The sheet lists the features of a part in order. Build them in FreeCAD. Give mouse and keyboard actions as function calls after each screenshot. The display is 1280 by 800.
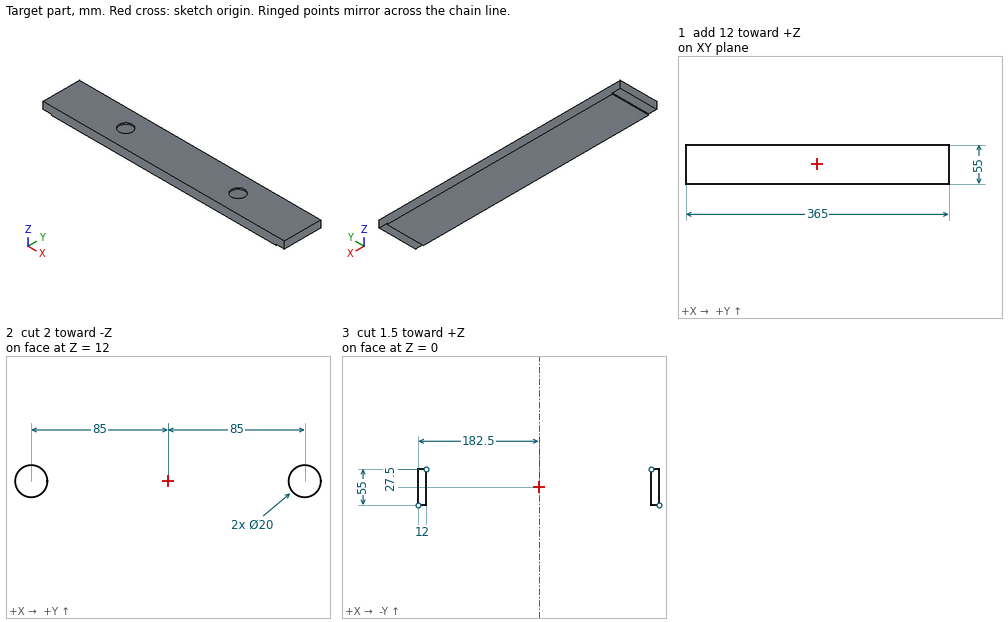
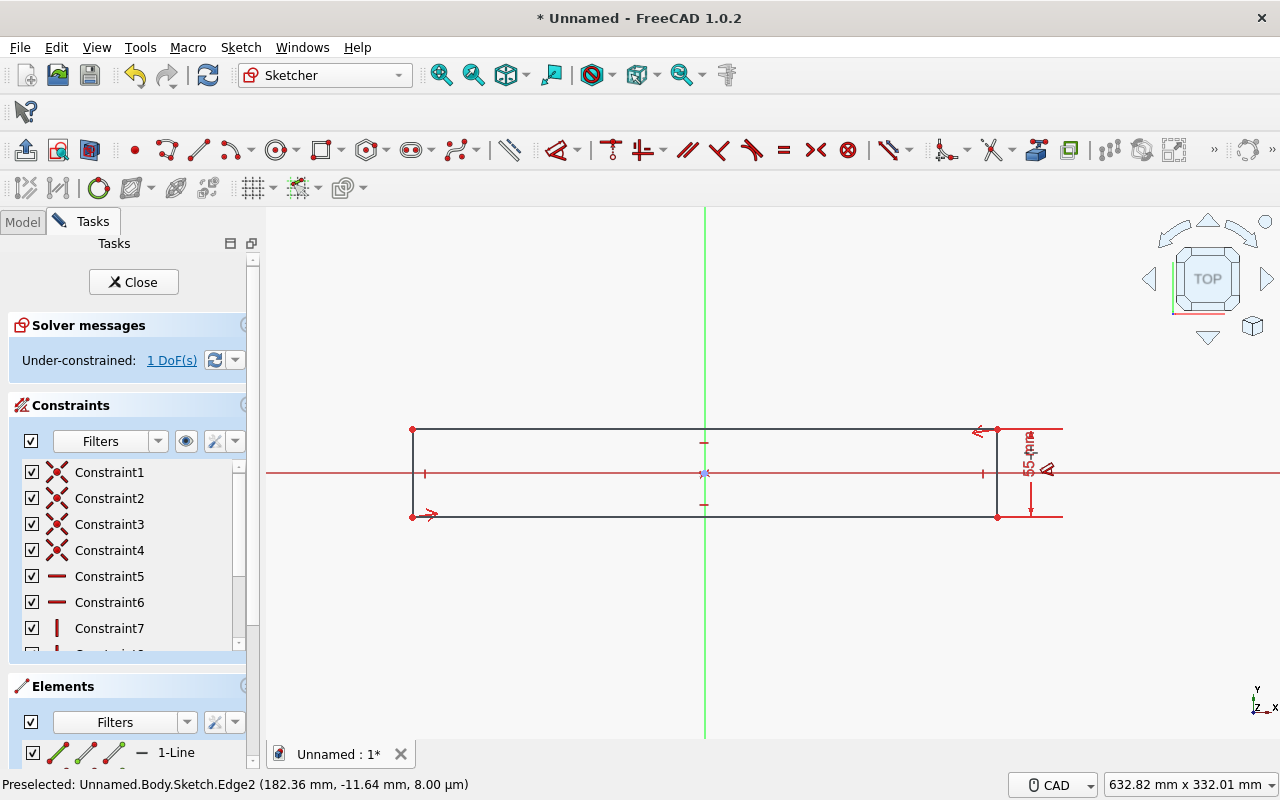
click(588, 517)
click(570, 551)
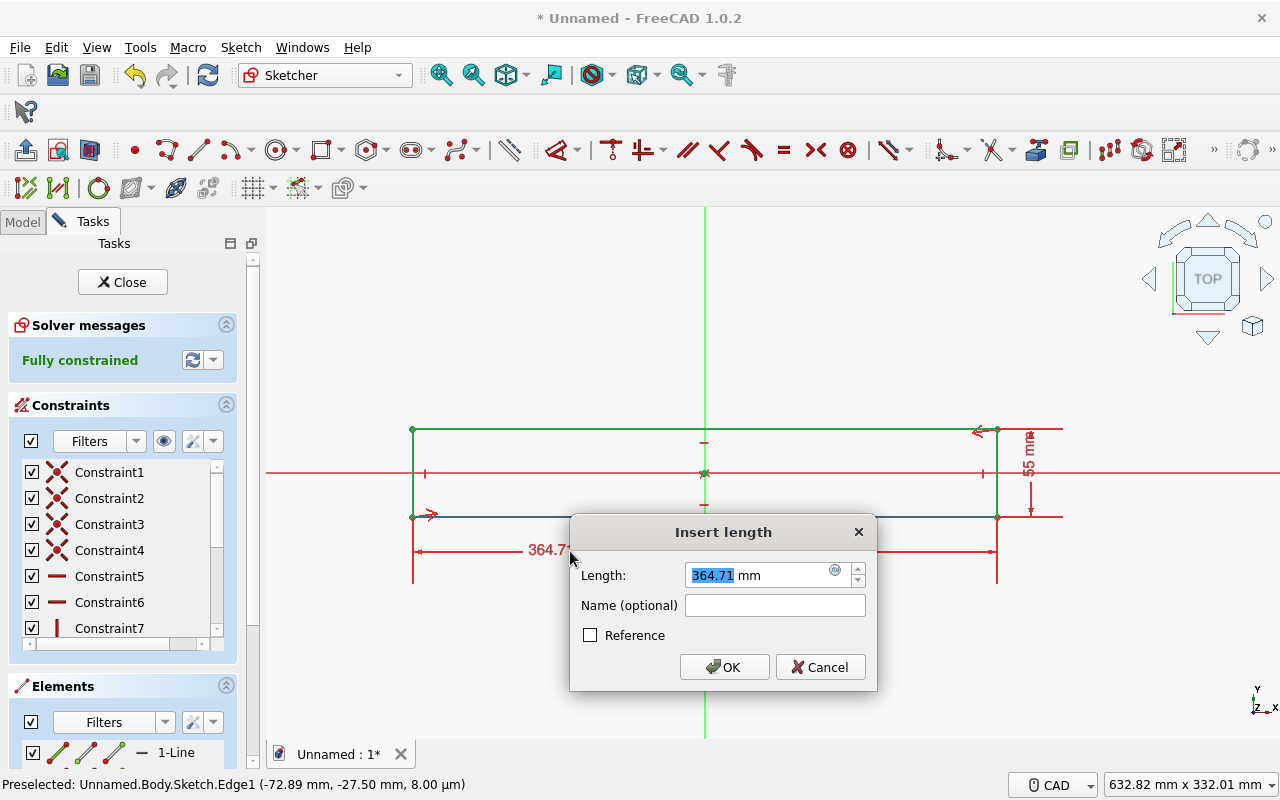
text(365)
key(Return)
key(Escape)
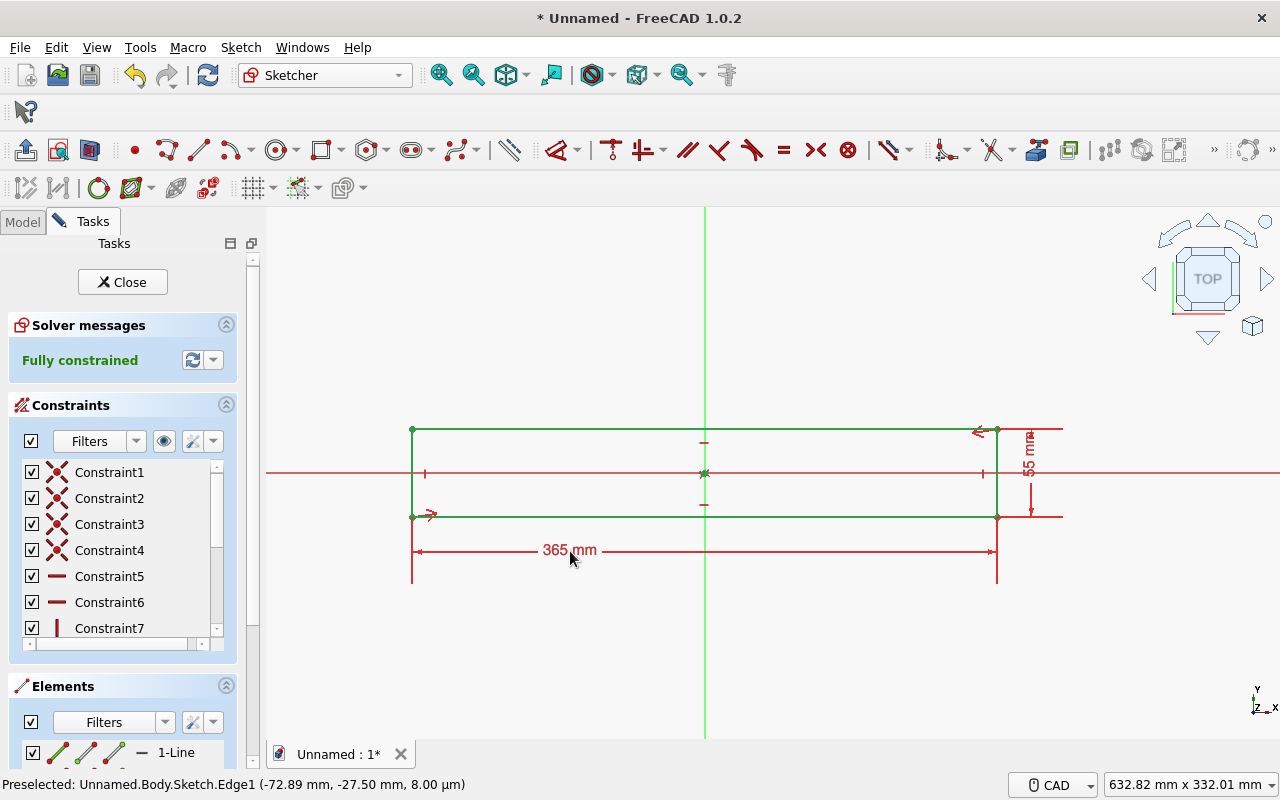
click(123, 282)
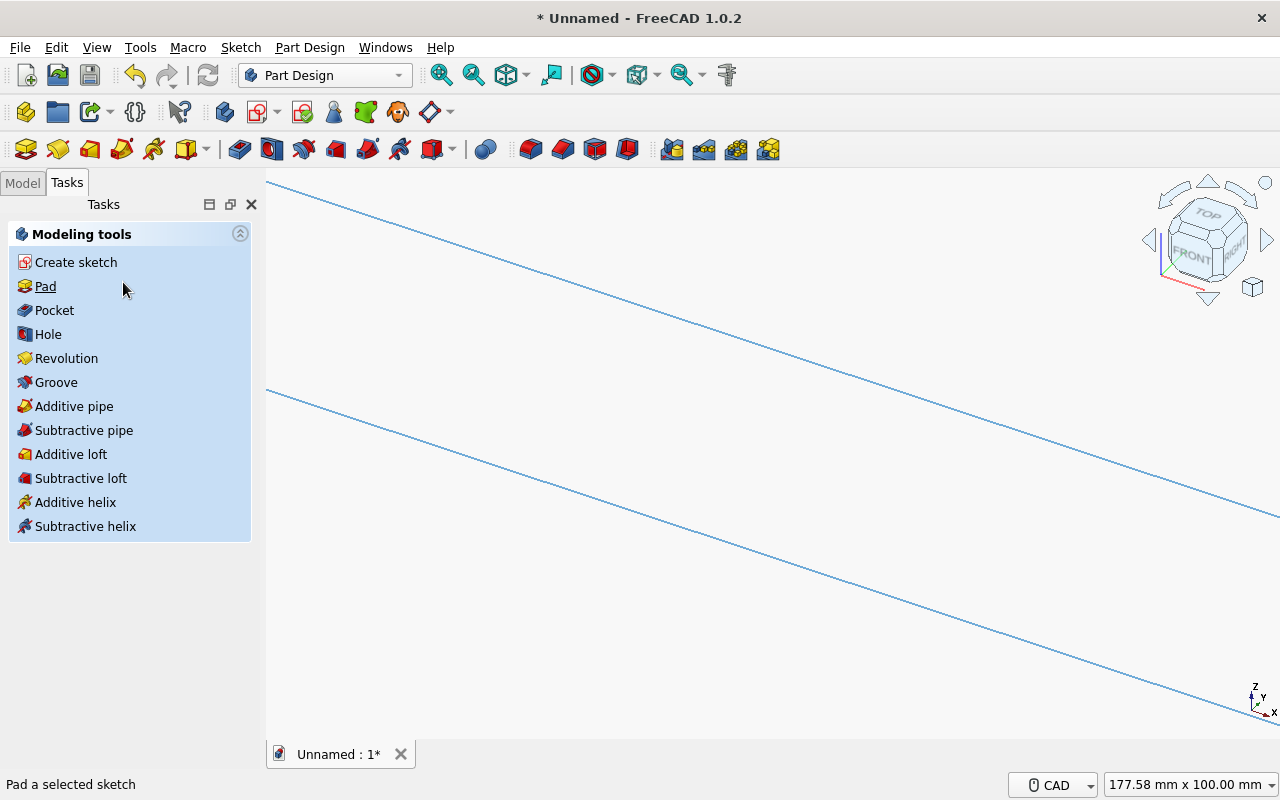
click(26, 150)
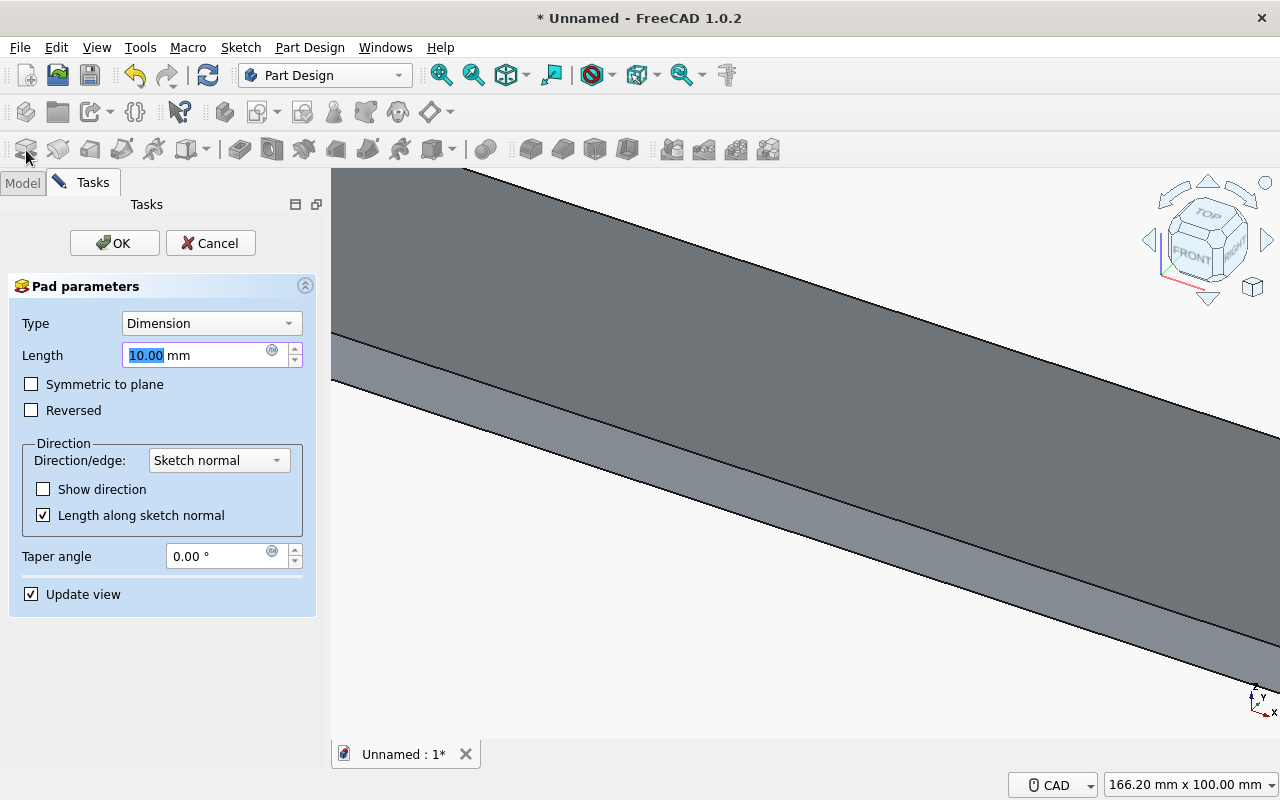
text(12)
key(Tab)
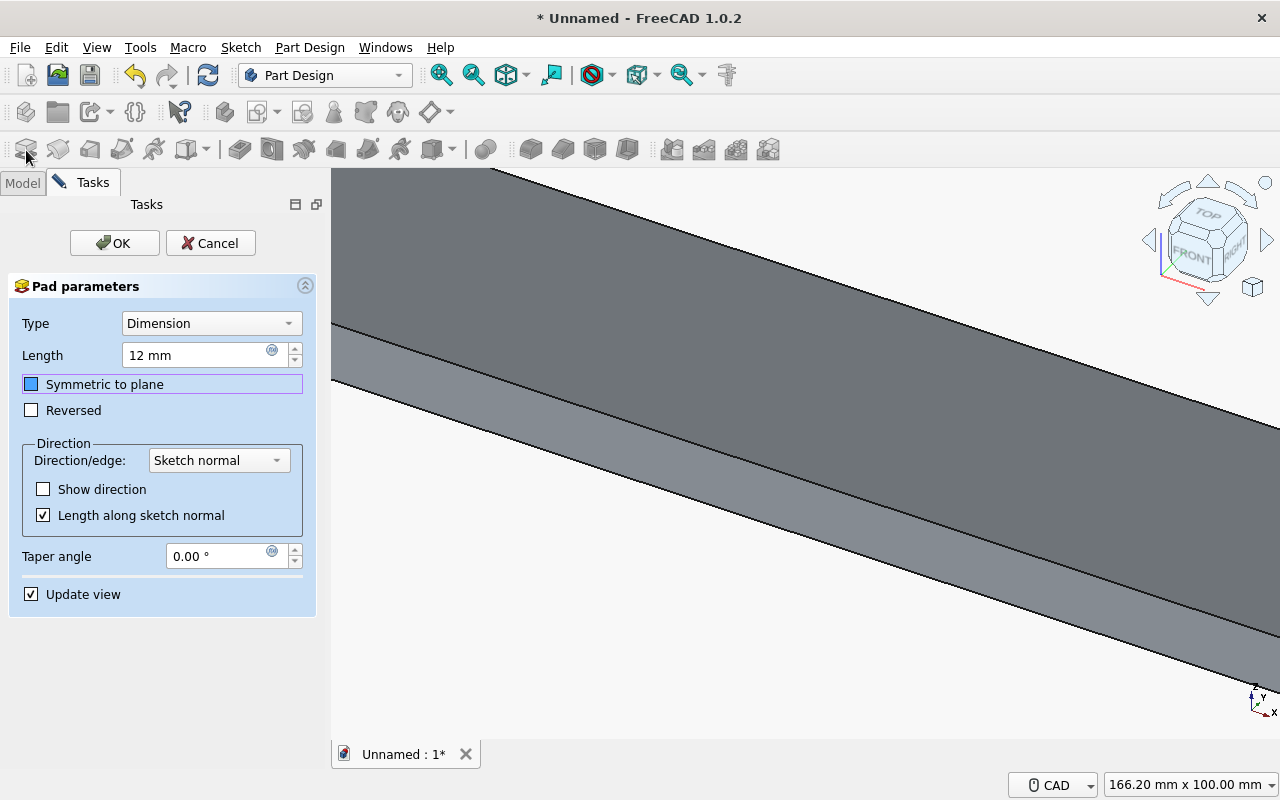
click(115, 243)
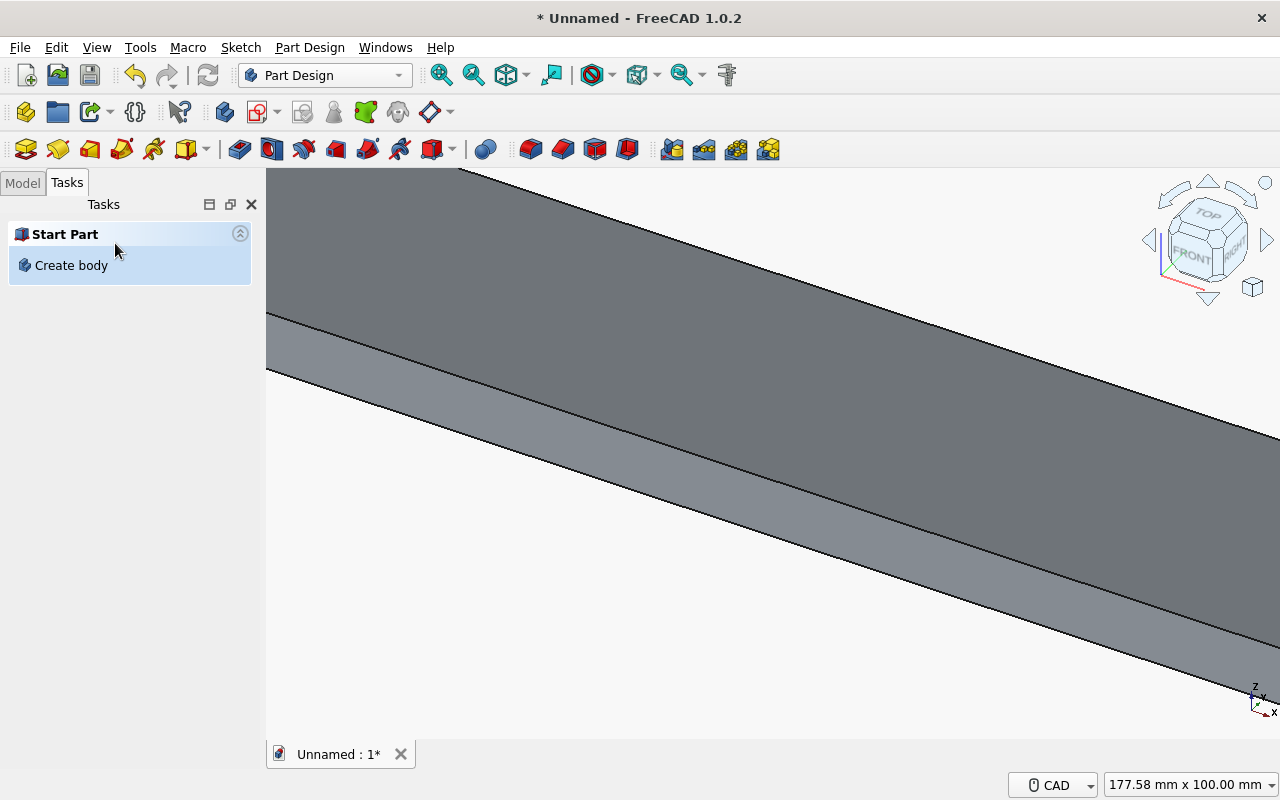
click(442, 76)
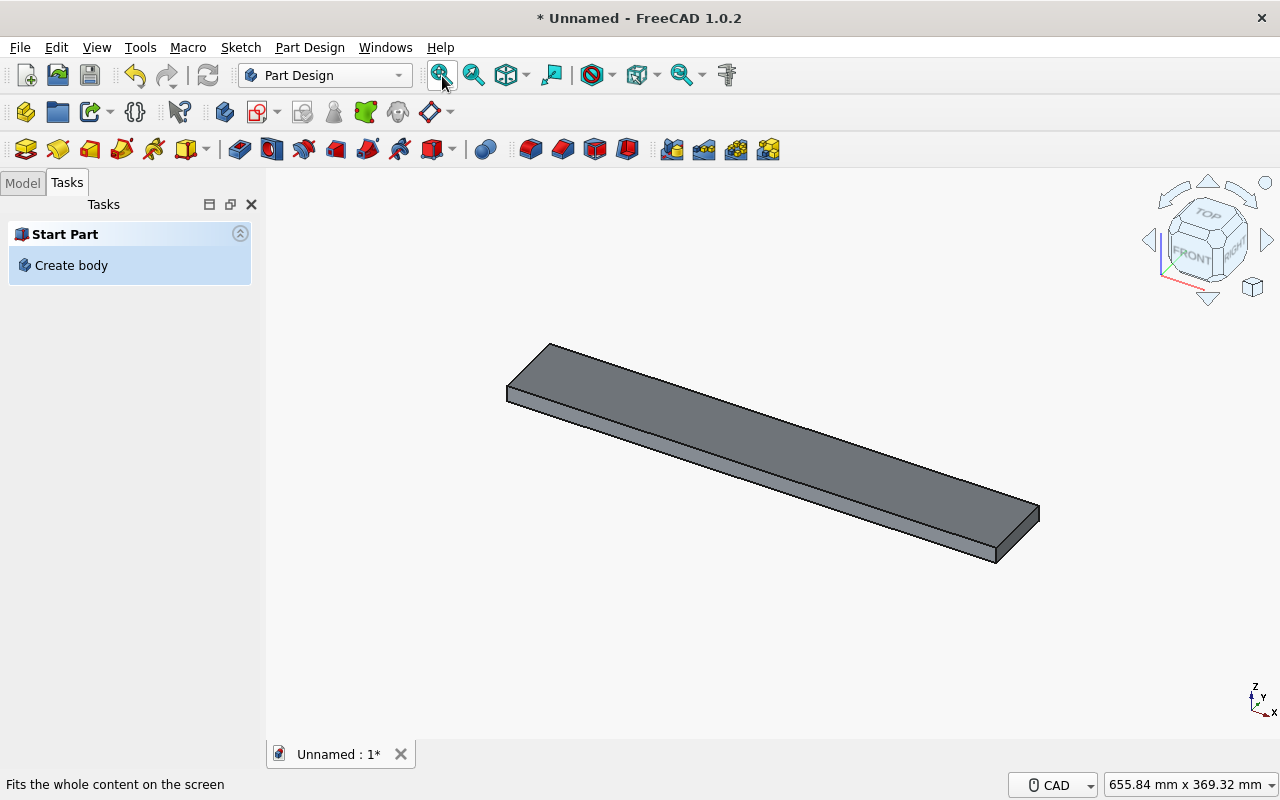
click(913, 491)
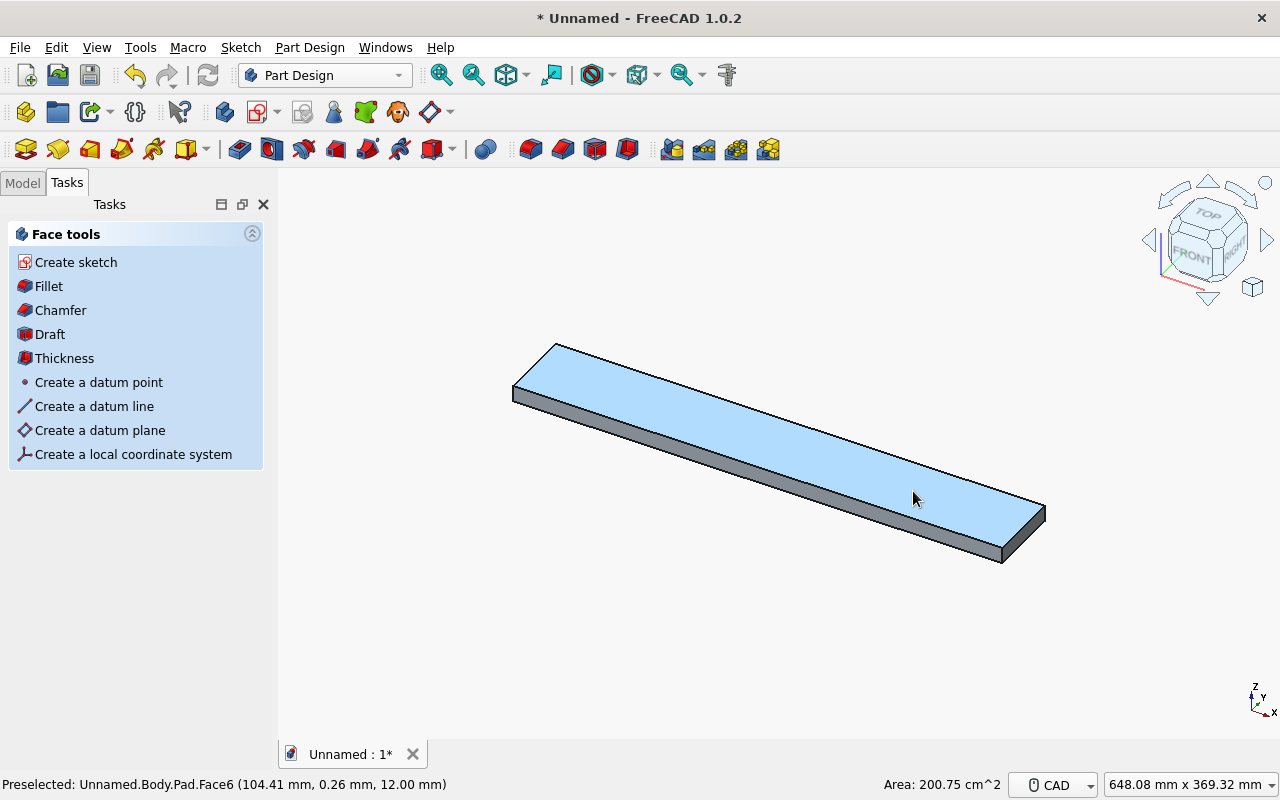
click(258, 112)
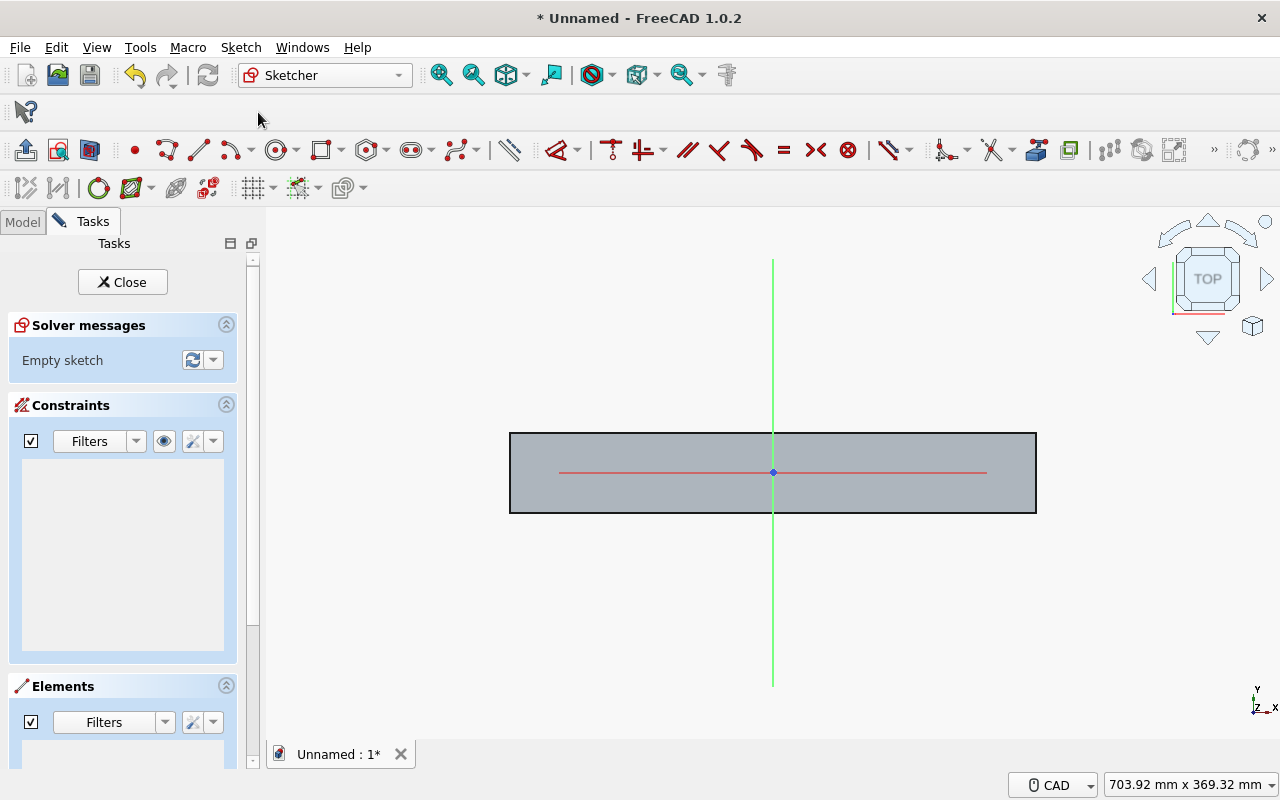
scroll(829, 473, up, 4)